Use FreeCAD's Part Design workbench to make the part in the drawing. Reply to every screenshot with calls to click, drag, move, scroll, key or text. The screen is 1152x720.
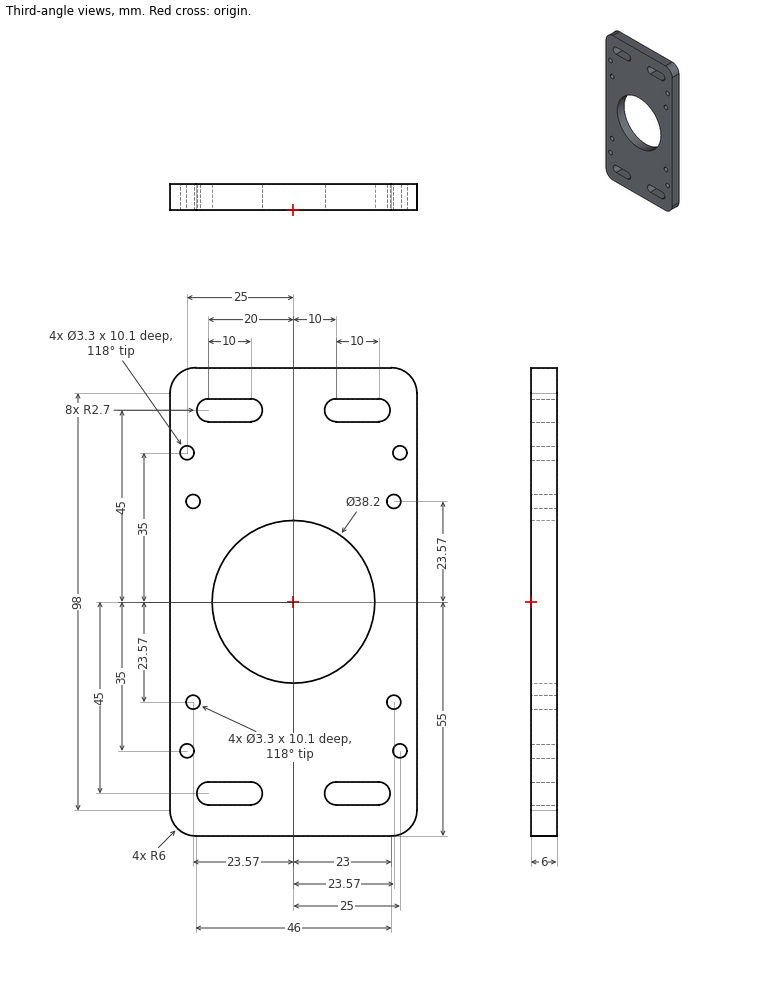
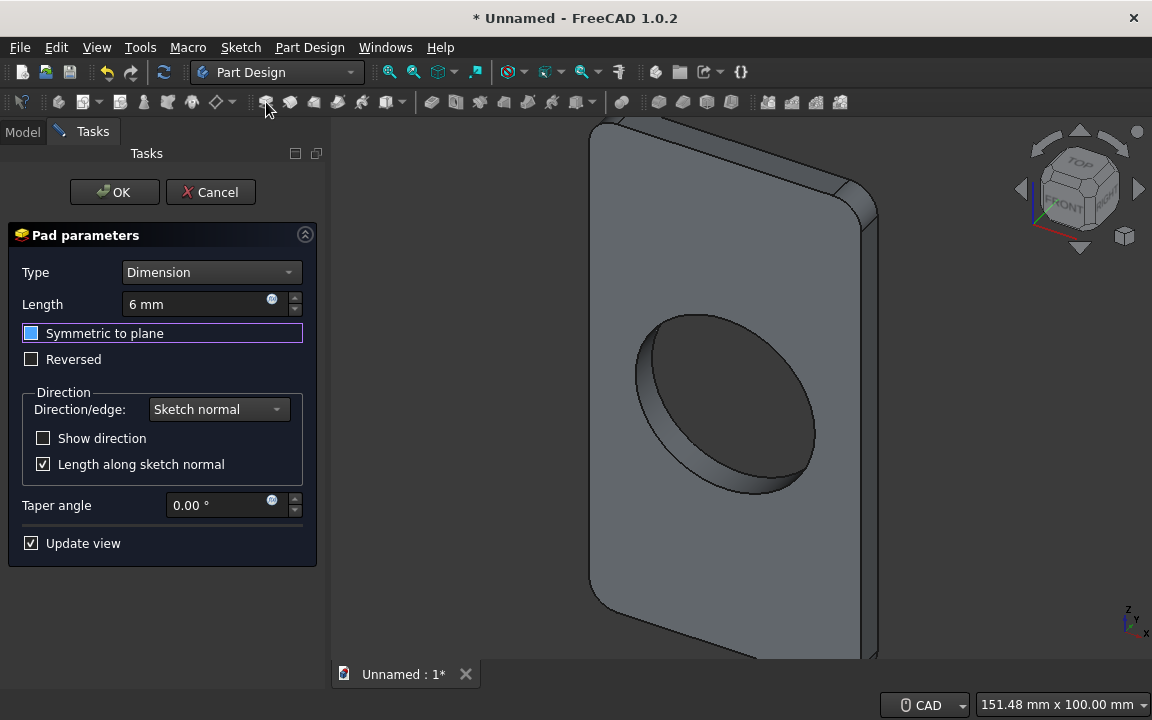
click(30, 359)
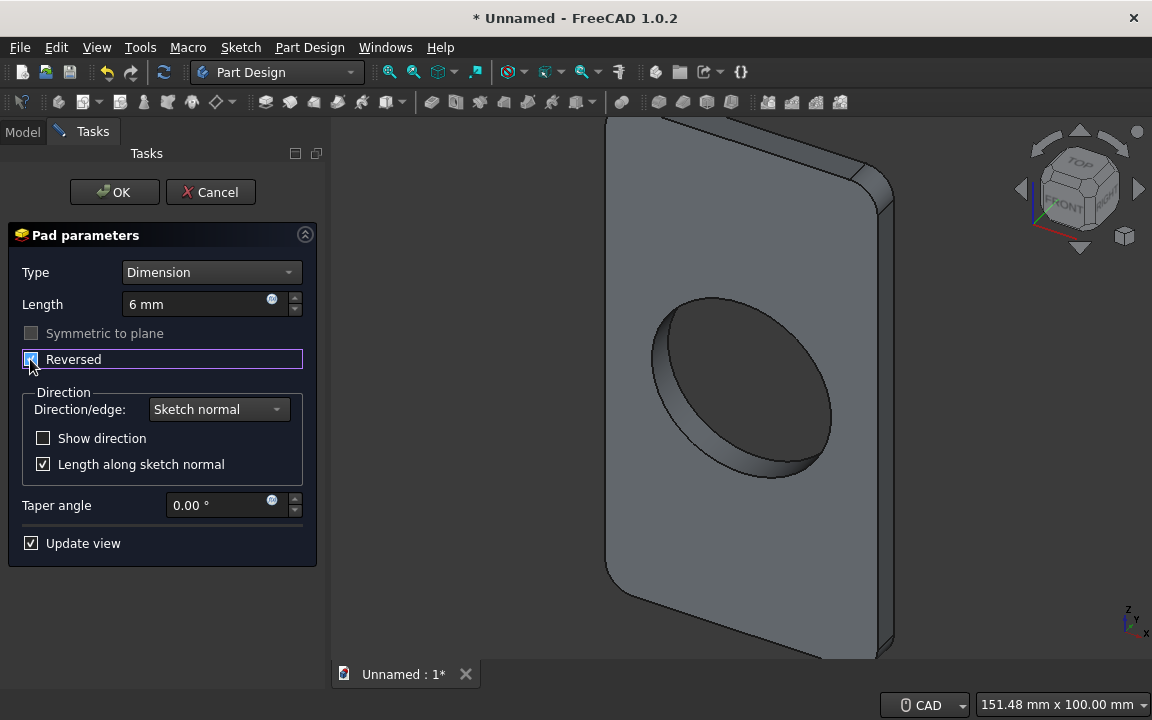
click(115, 192)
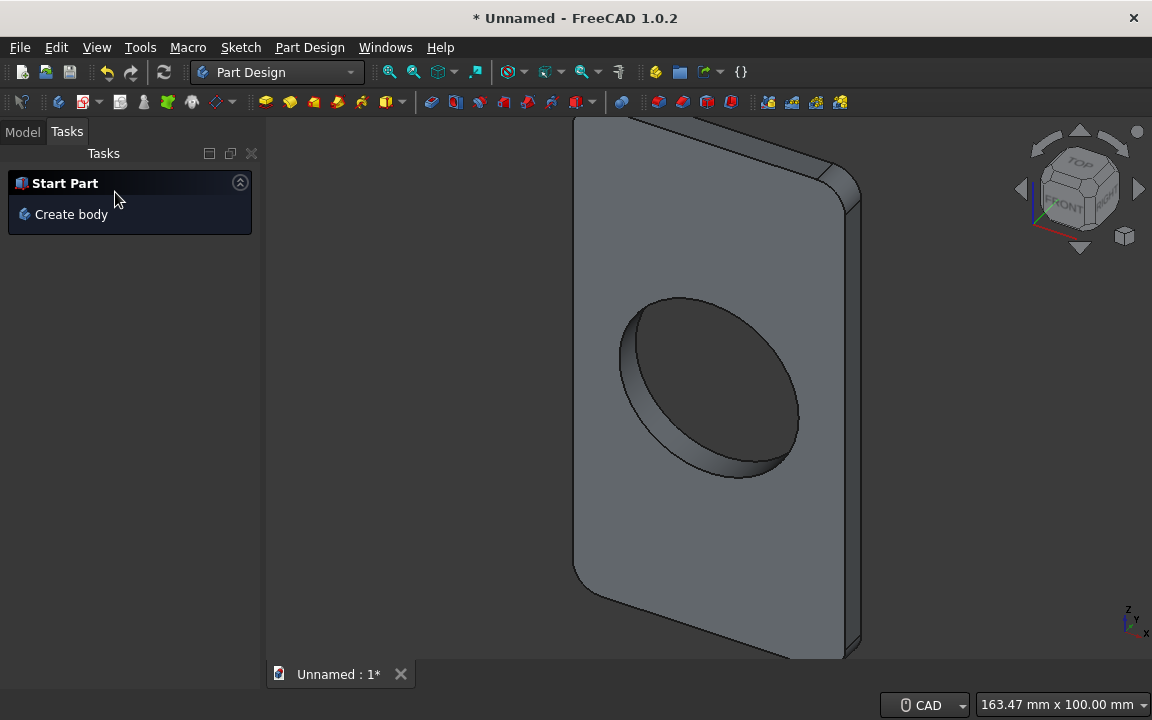
click(390, 72)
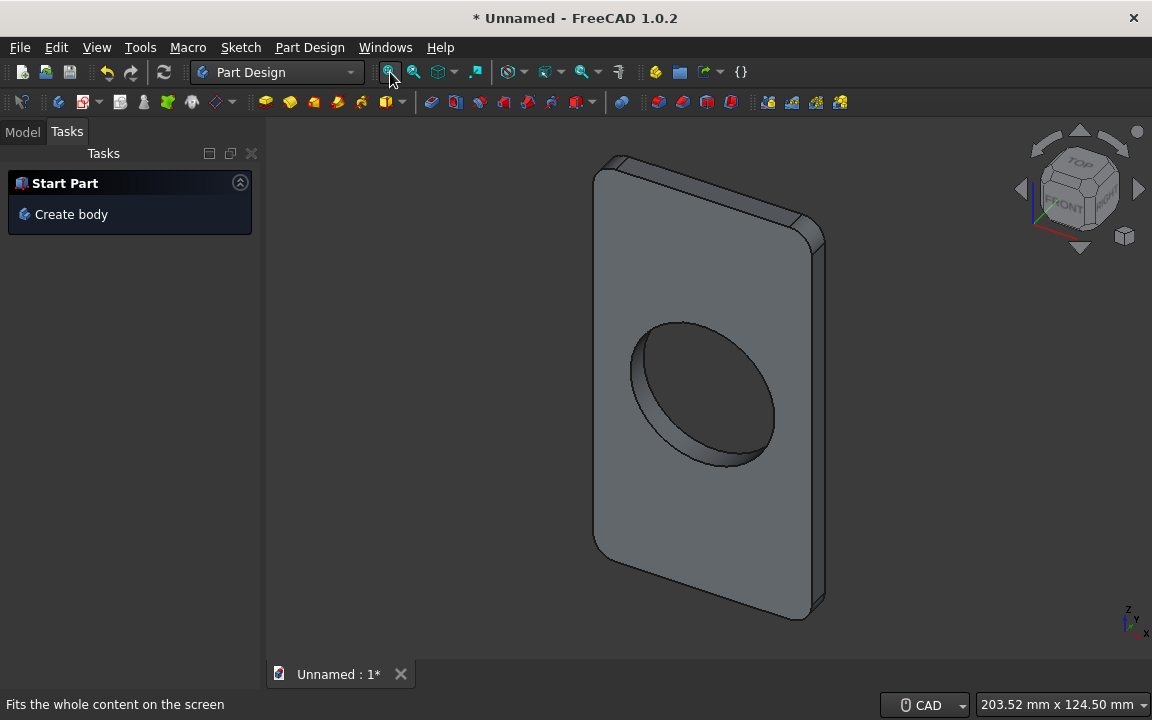
key(4)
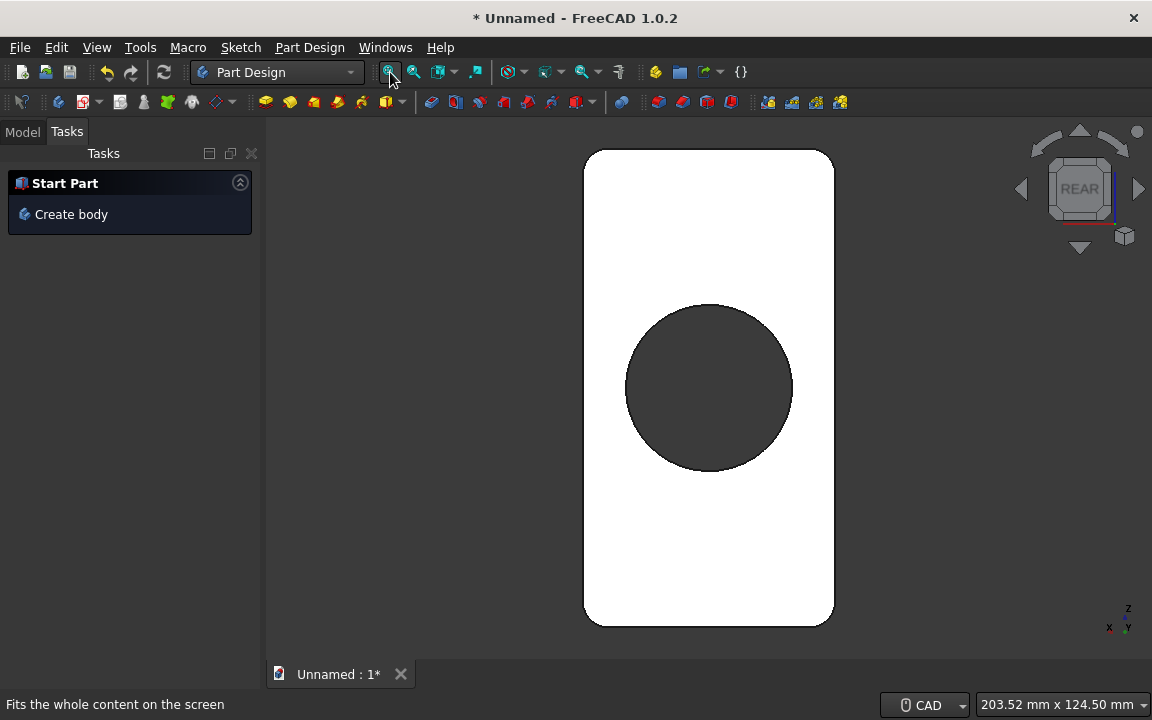
click(673, 250)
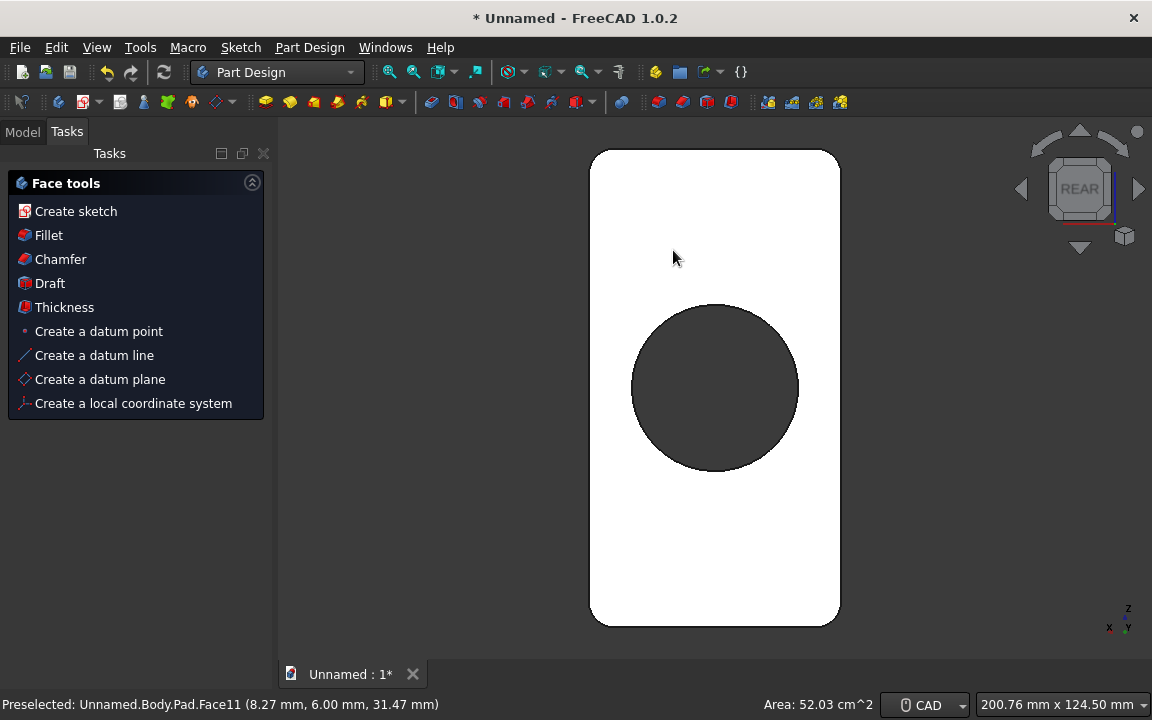
click(84, 102)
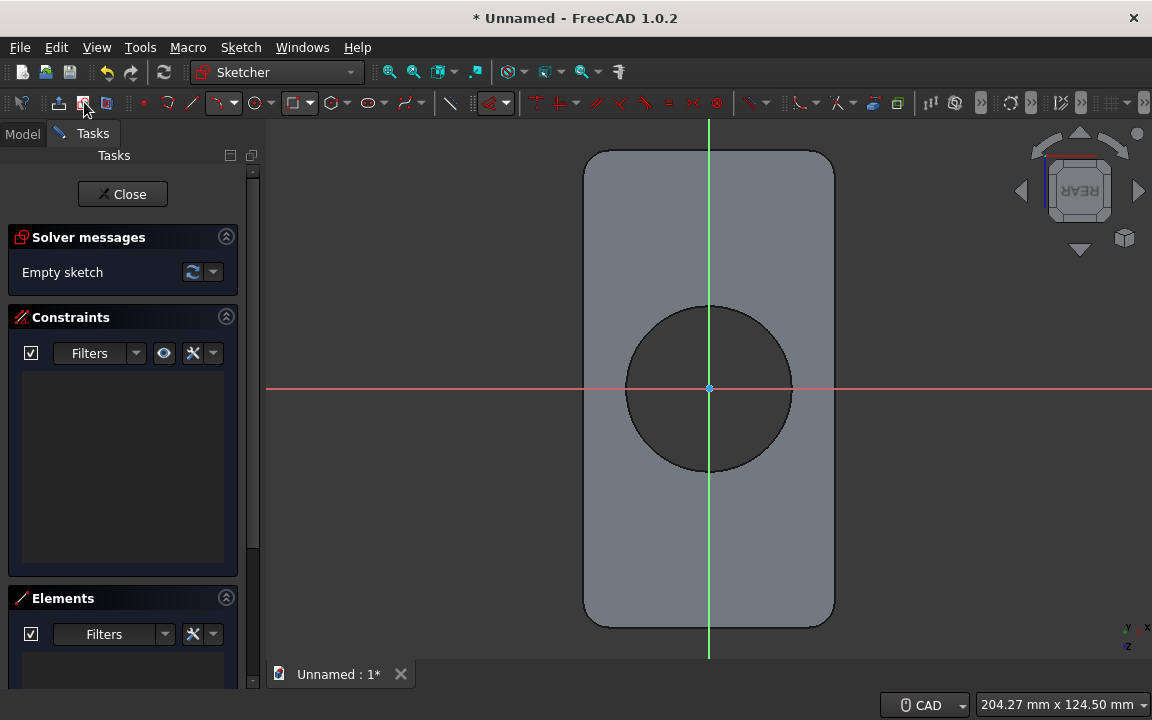
scroll(848, 389, up, 2)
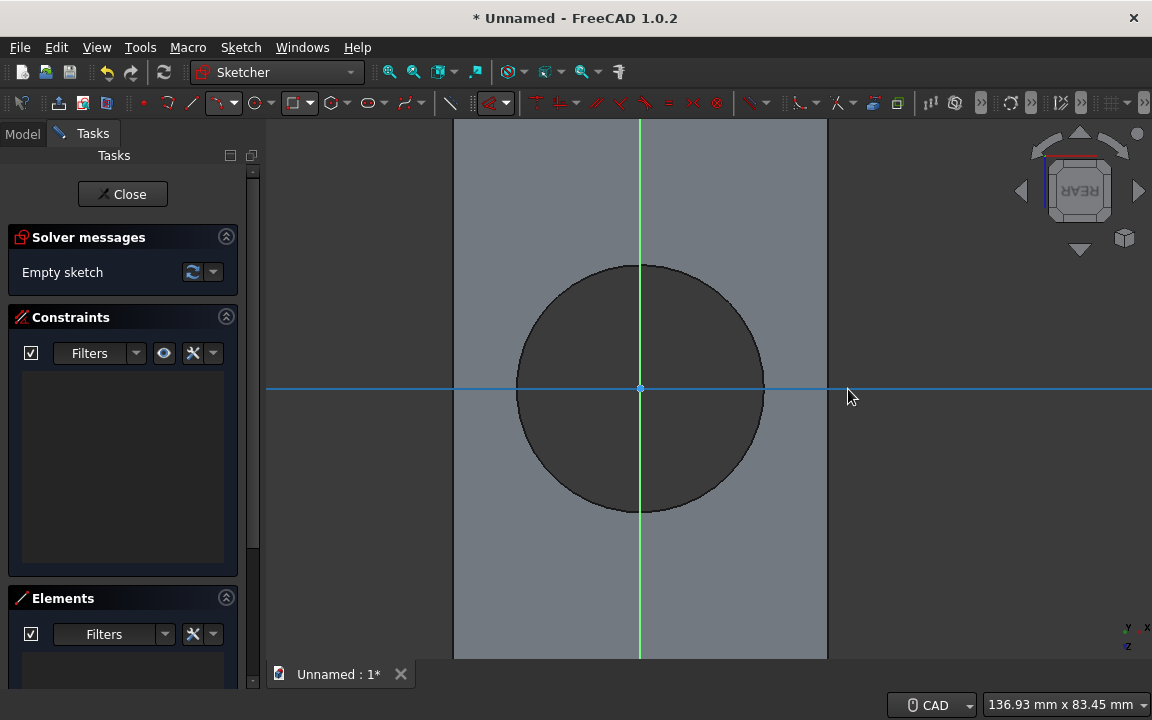
key(g)
key(c)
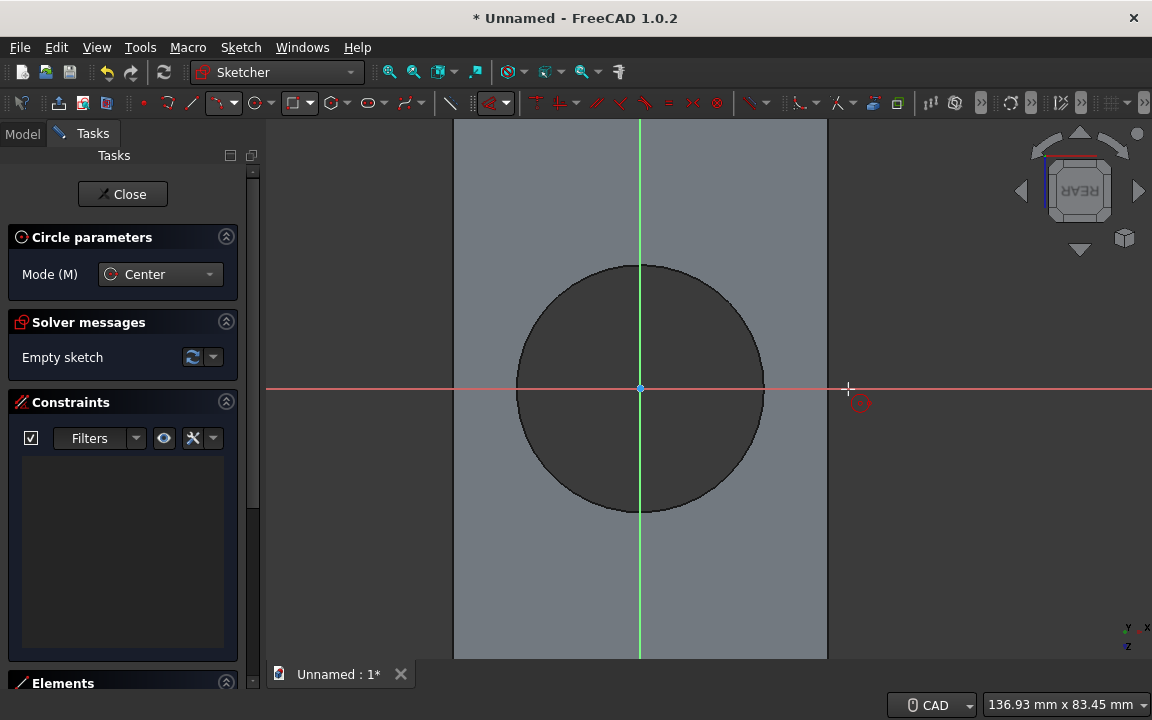
scroll(488, 236, up, 4)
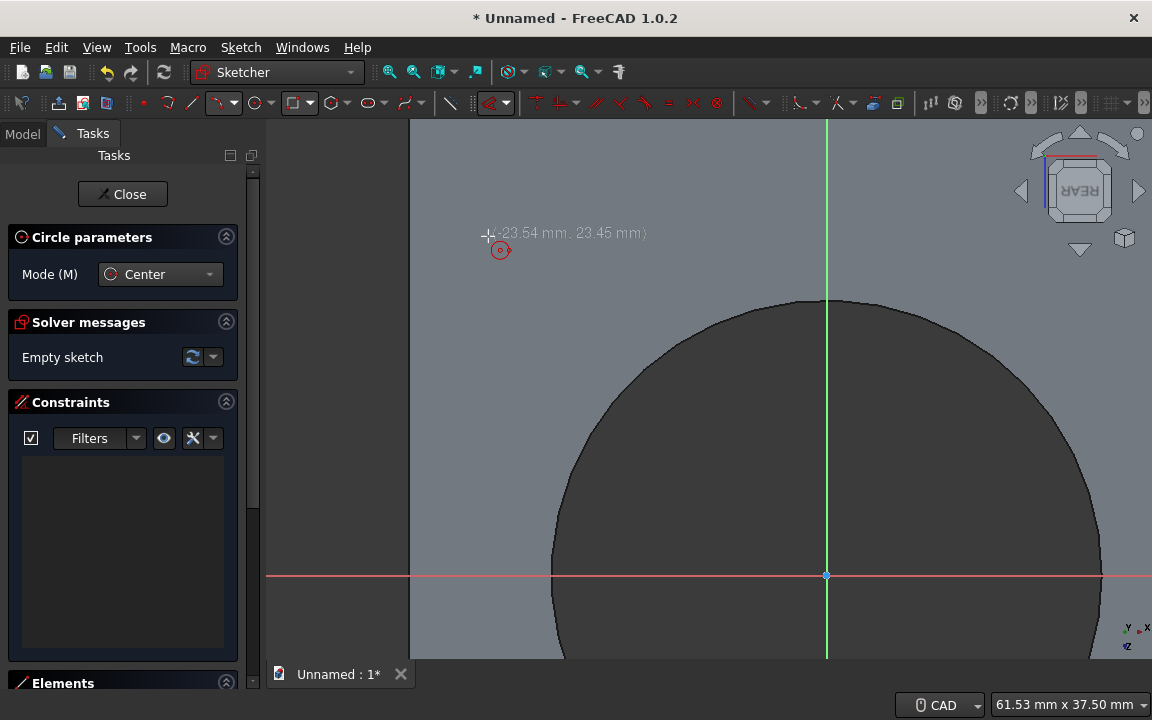
click(487, 236)
move(504, 219)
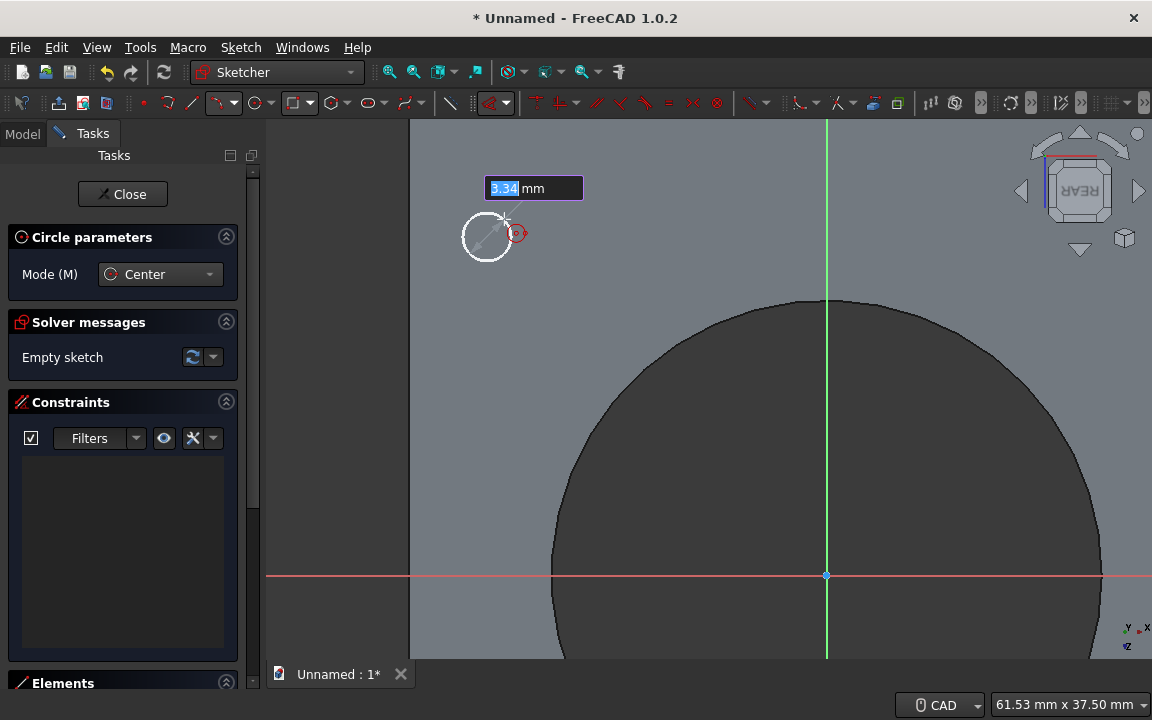
text(3.3)
key(Return)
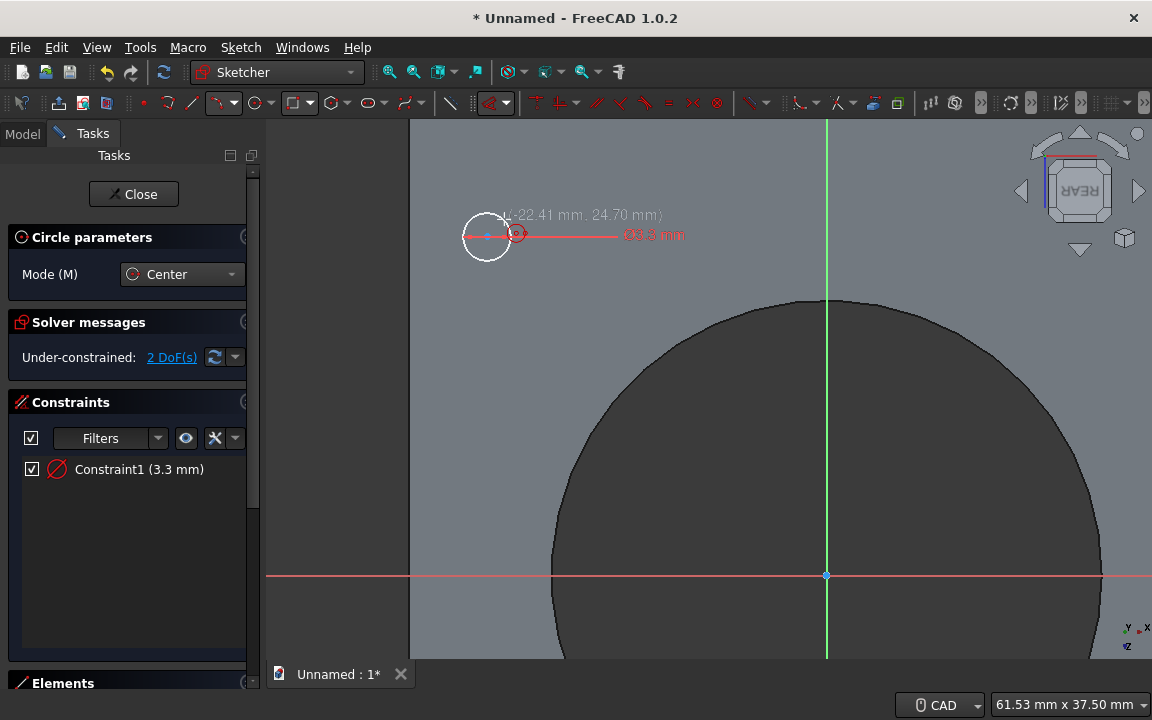
scroll(489, 237, down, 4)